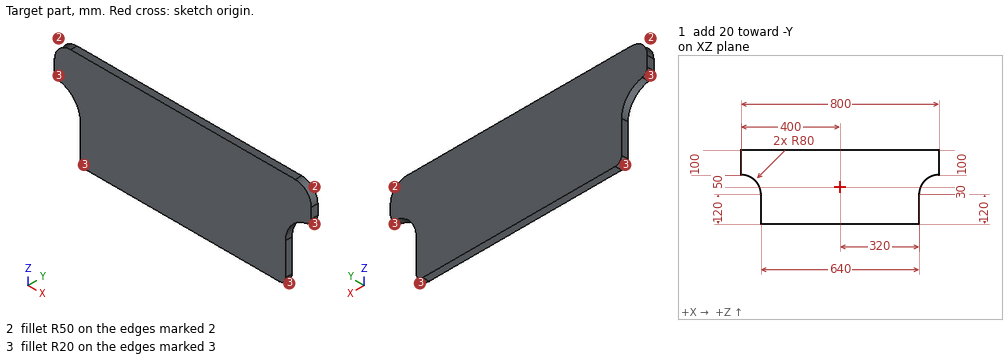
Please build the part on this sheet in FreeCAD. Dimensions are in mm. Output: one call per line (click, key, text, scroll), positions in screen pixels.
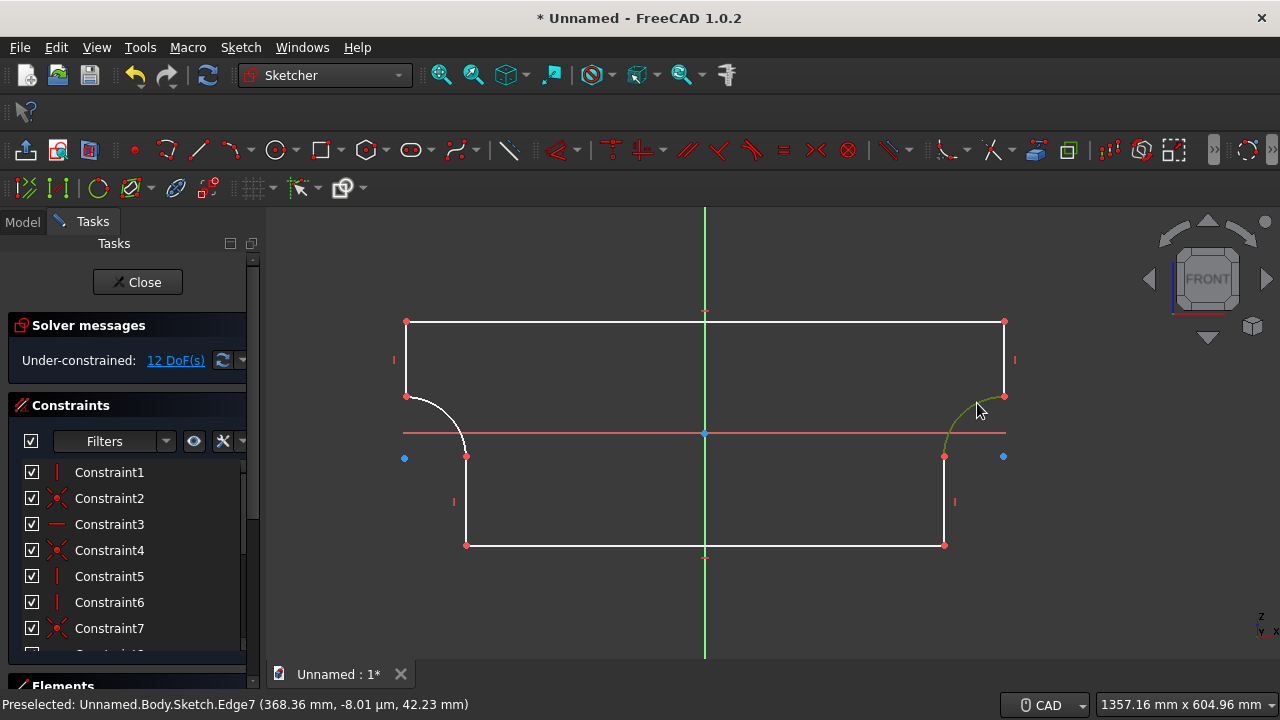
click(459, 430)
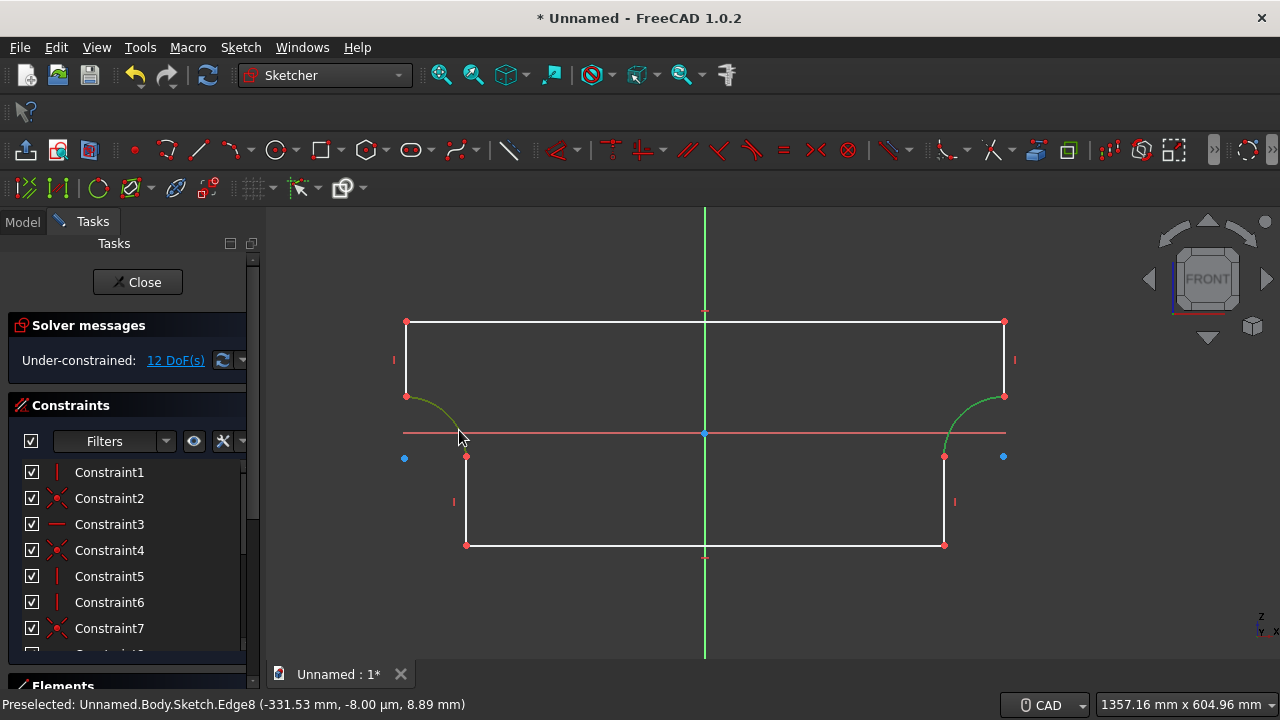
key(e)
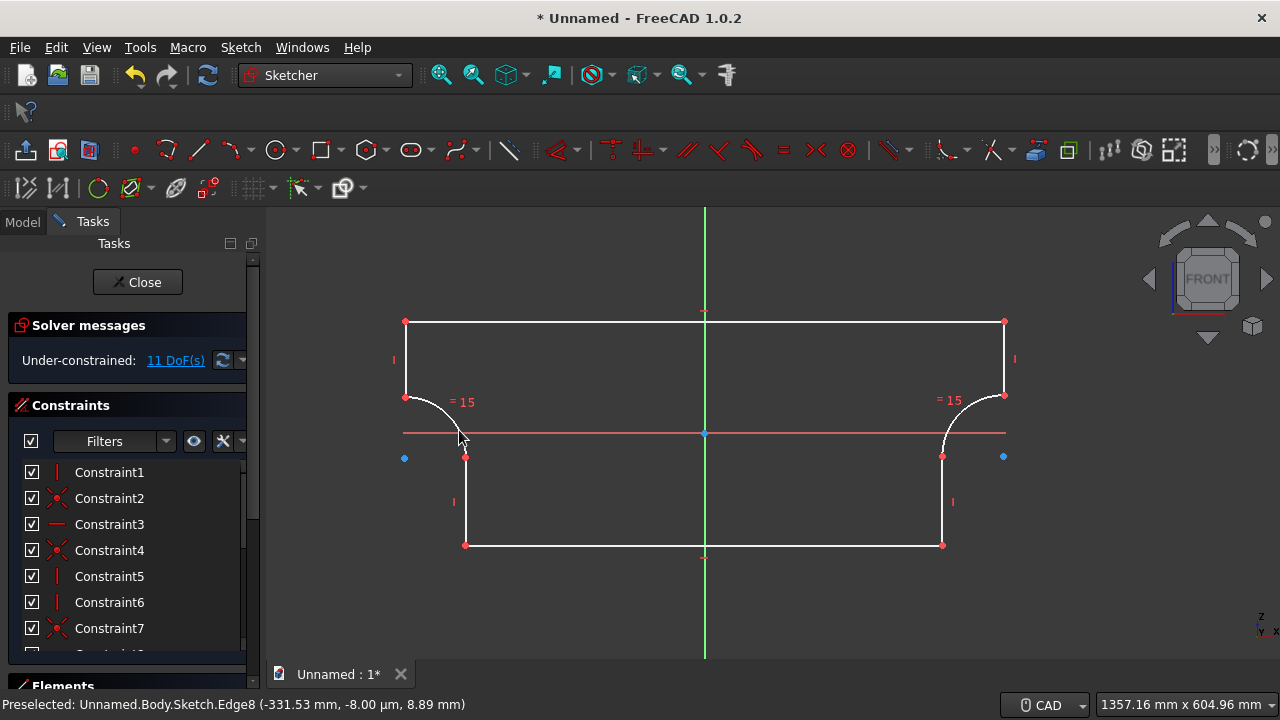
click(976, 402)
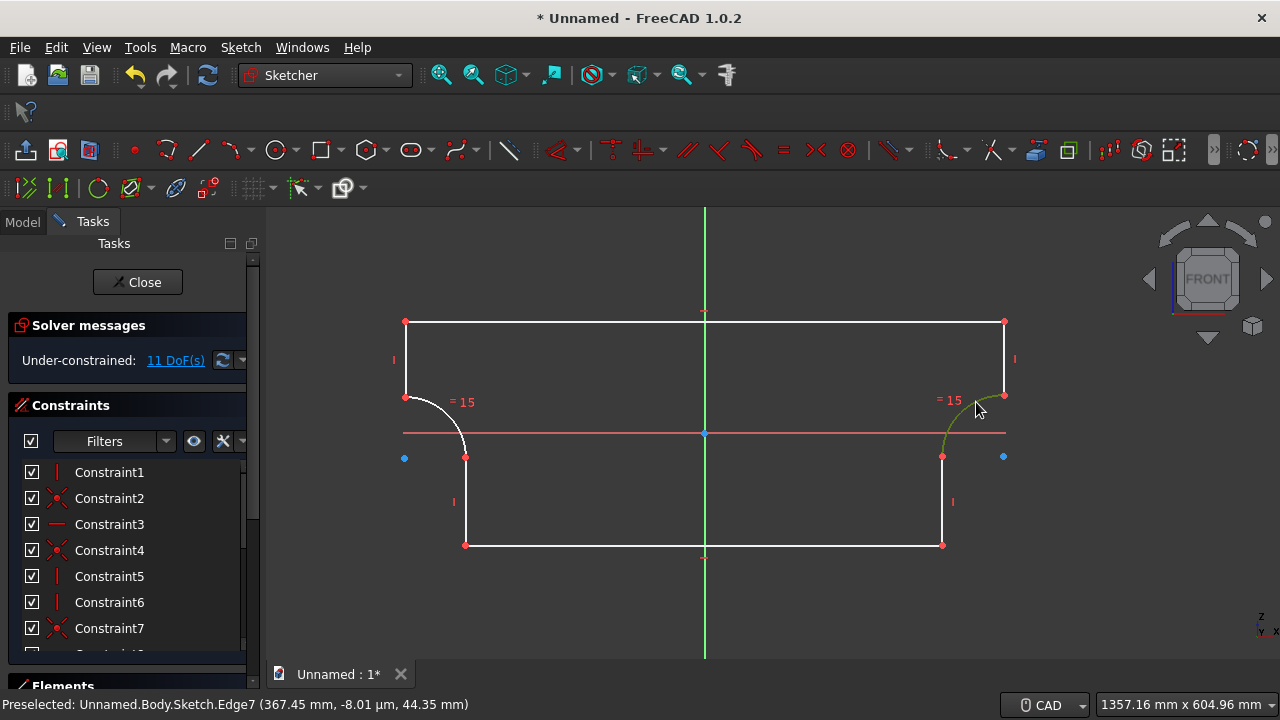
key(k)
key(r)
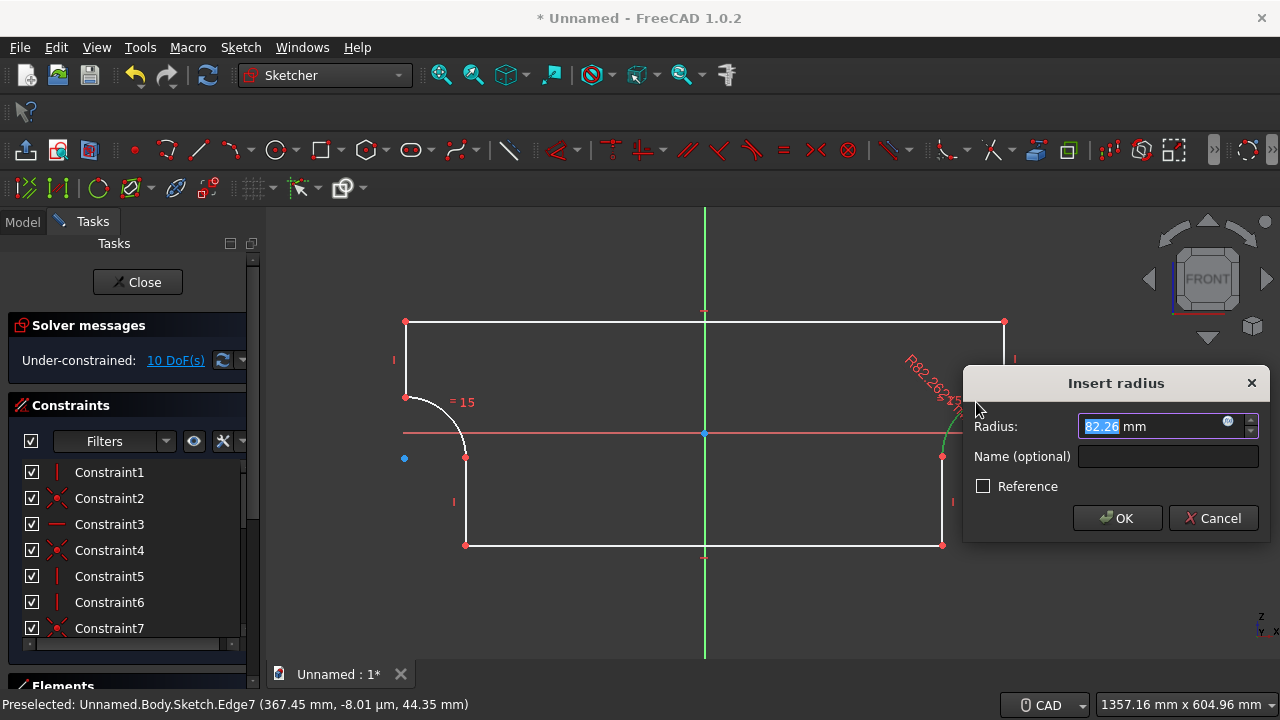
text(80)
key(Return)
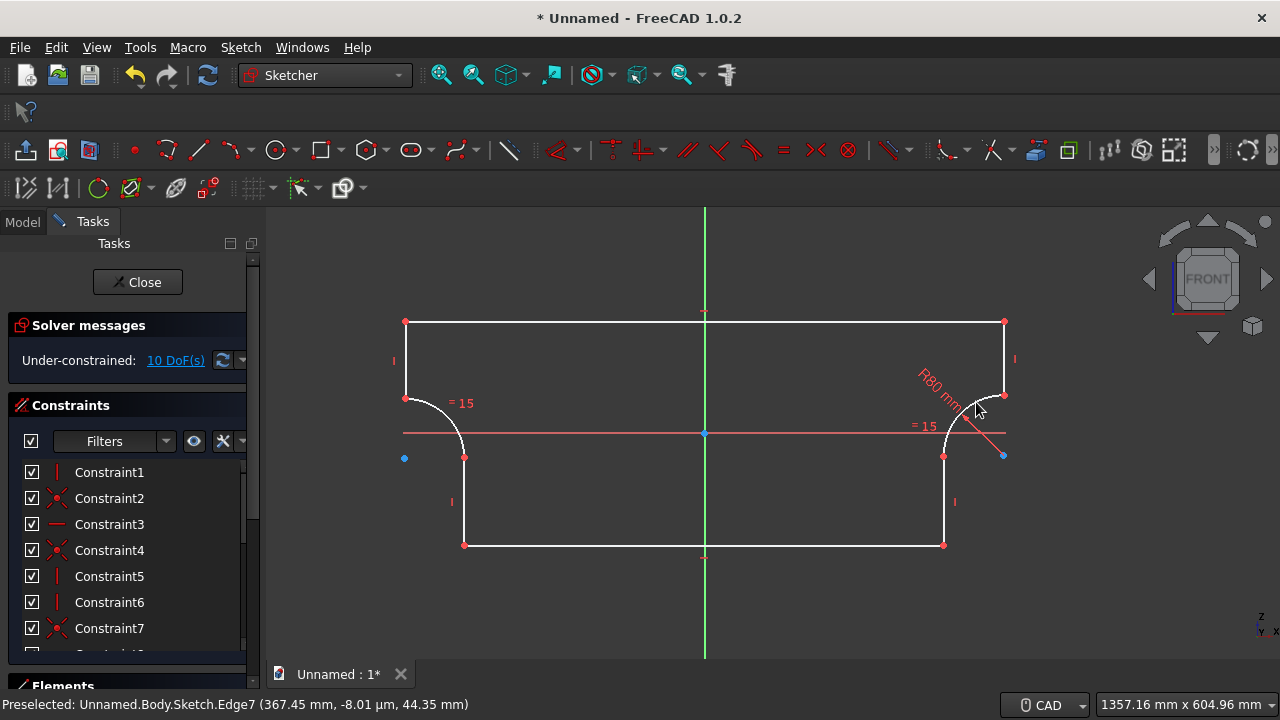
click(406, 376)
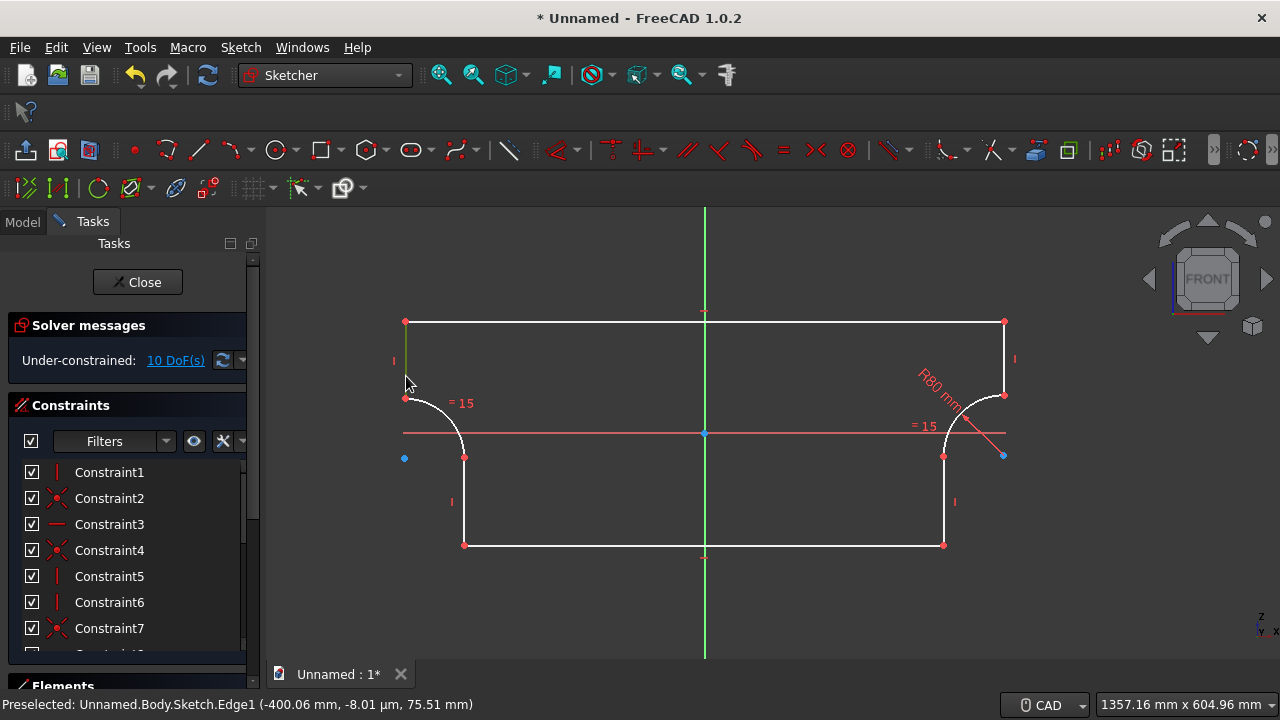
key(i)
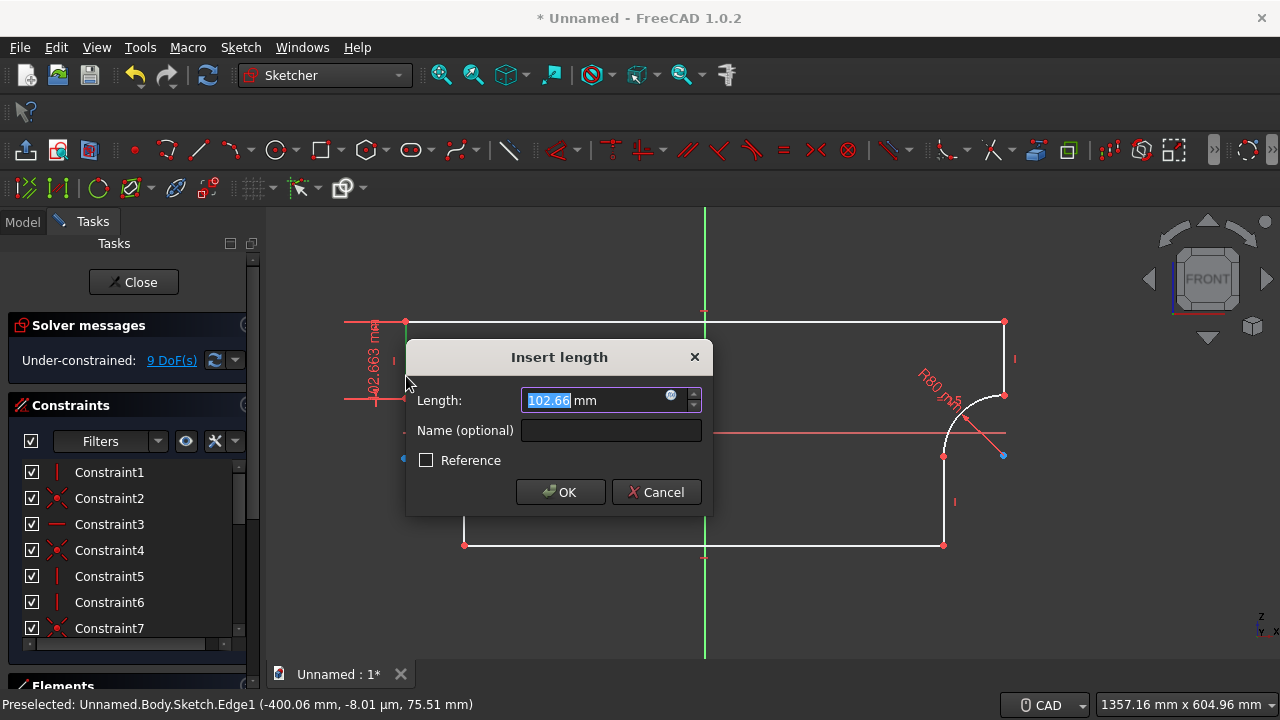
text(100)
key(Return)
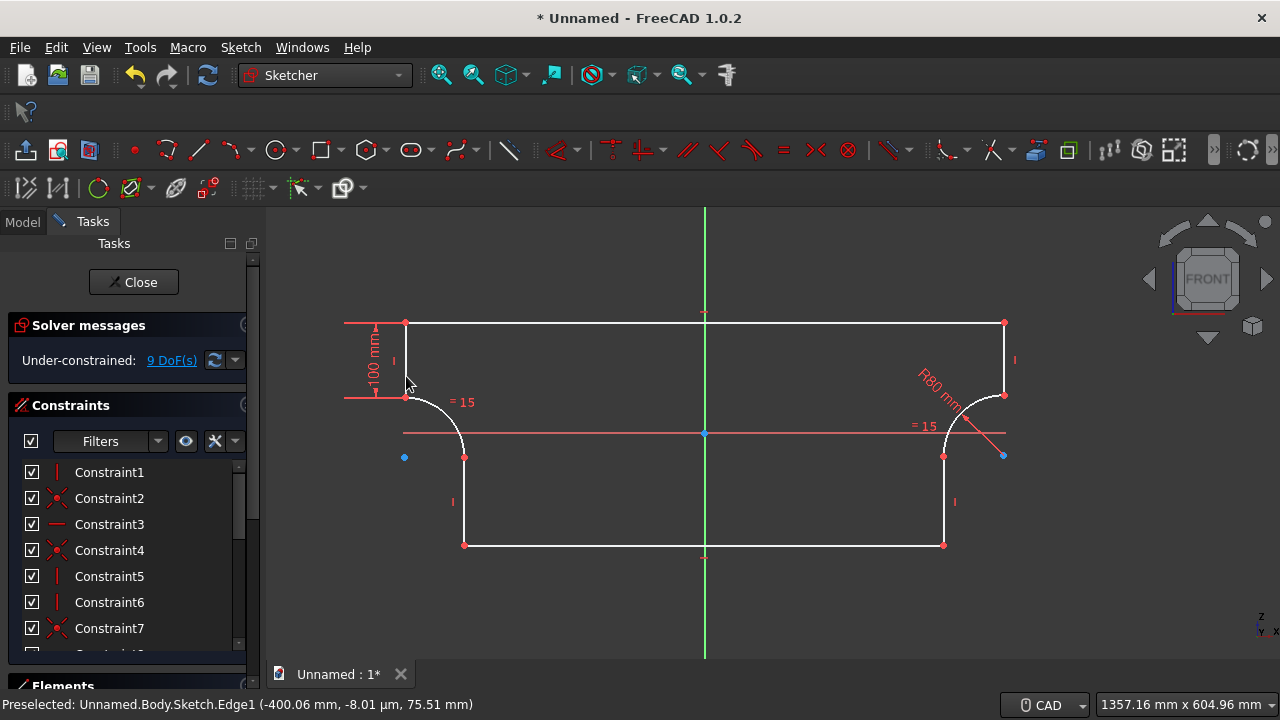
click(585, 323)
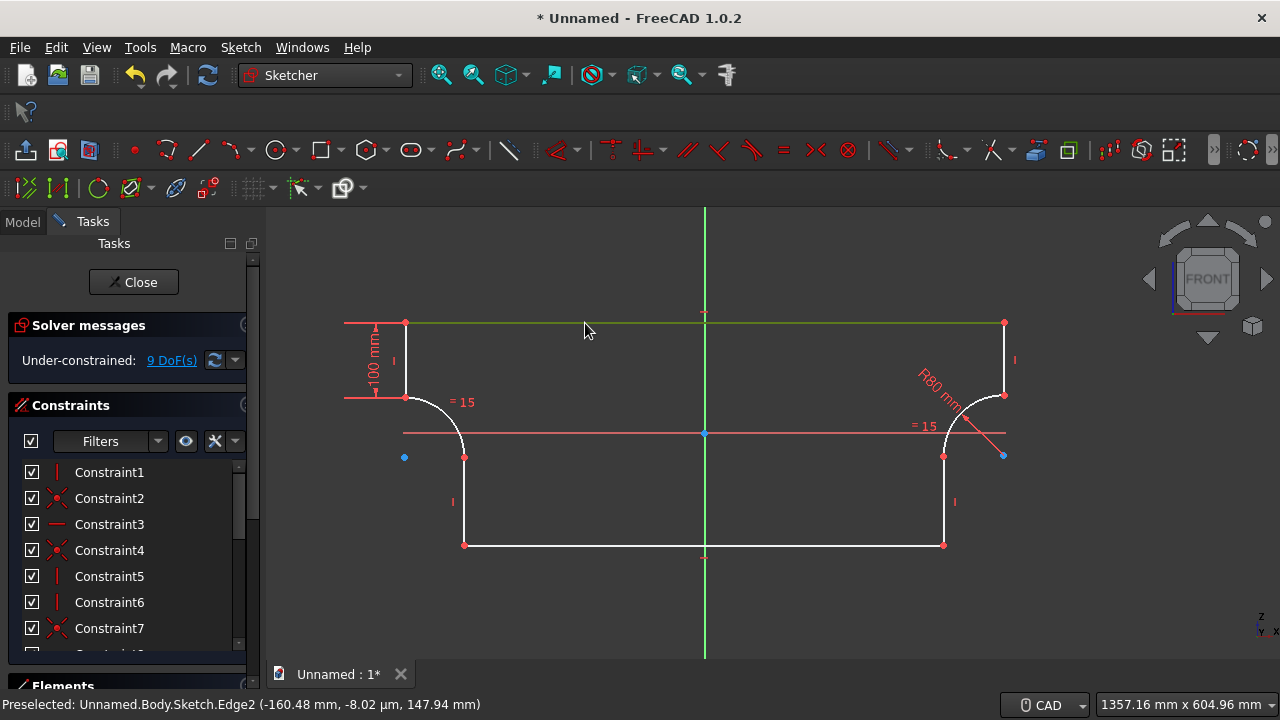
key(l)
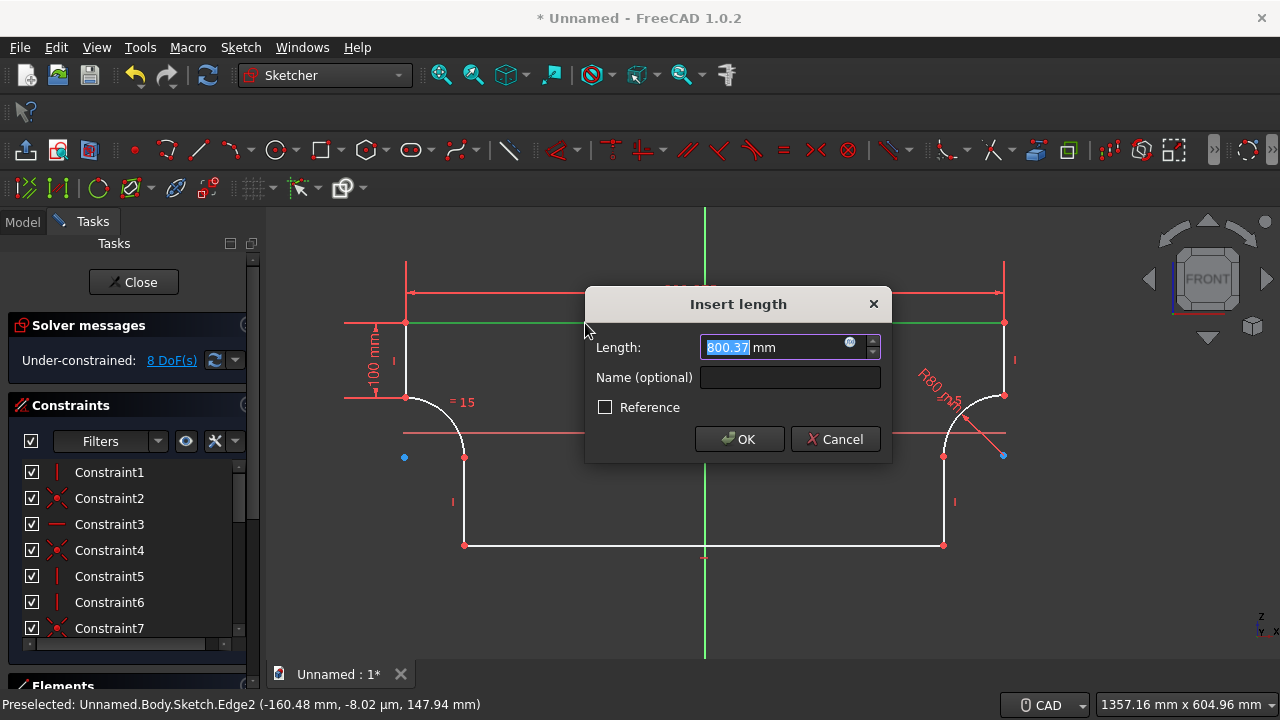
text(800)
key(Return)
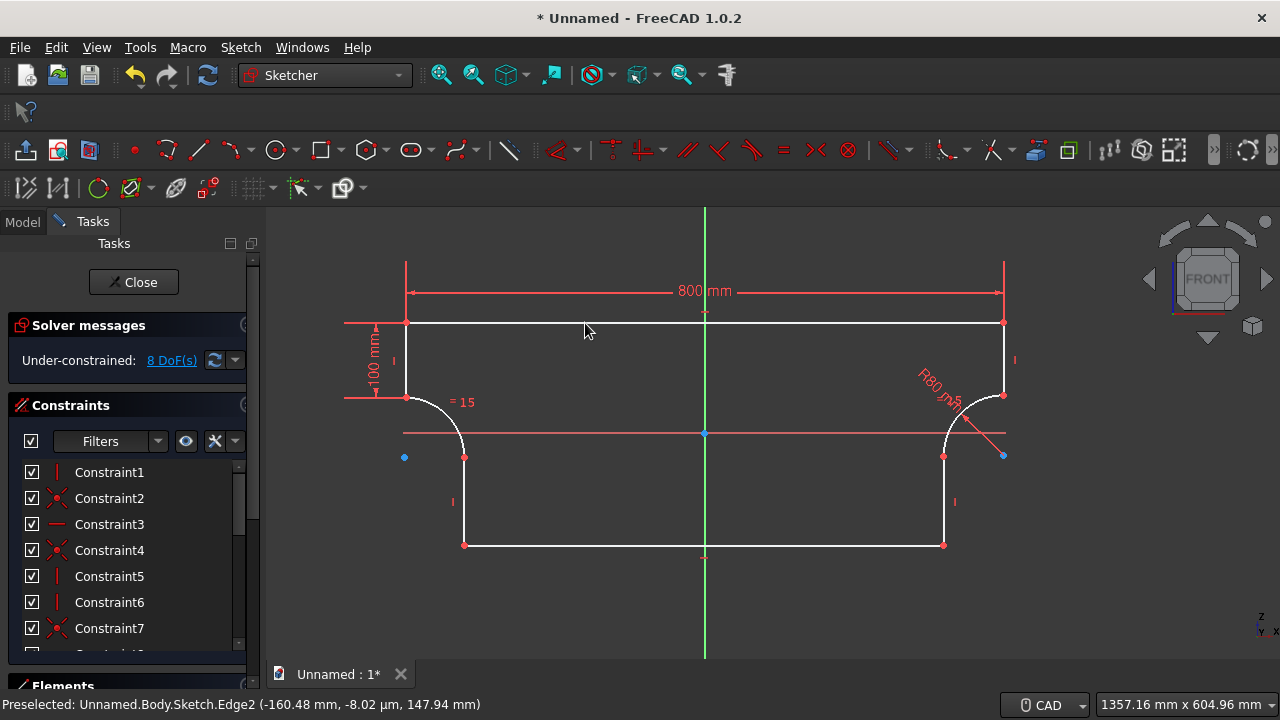
click(1004, 345)